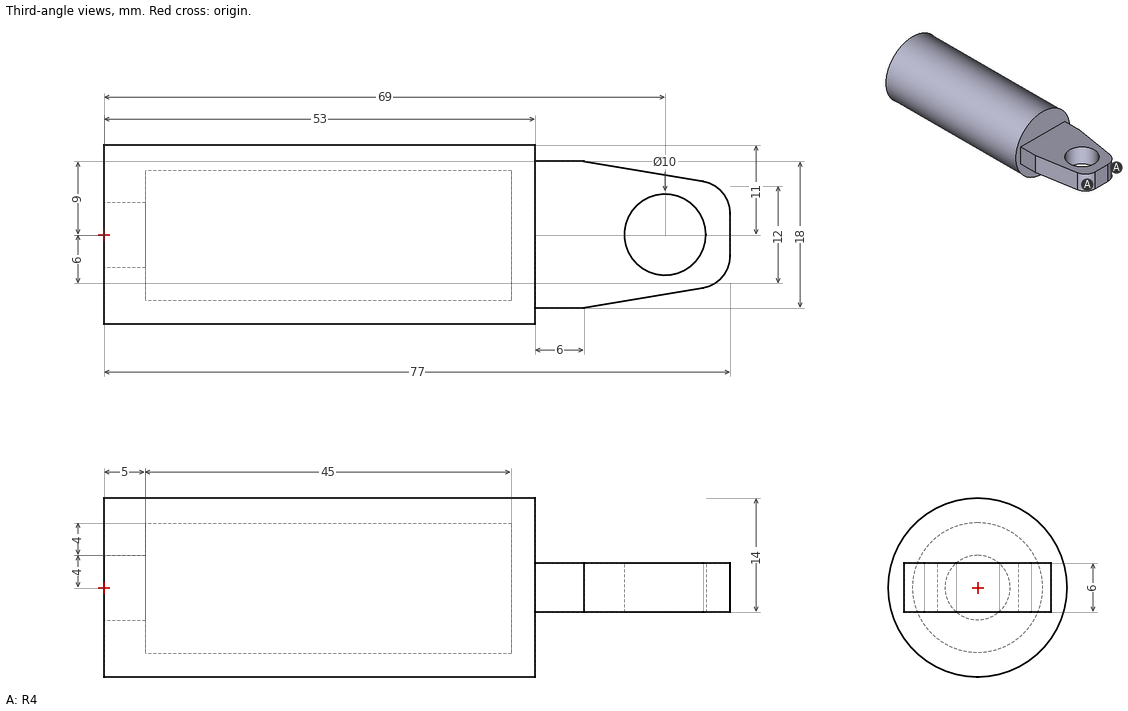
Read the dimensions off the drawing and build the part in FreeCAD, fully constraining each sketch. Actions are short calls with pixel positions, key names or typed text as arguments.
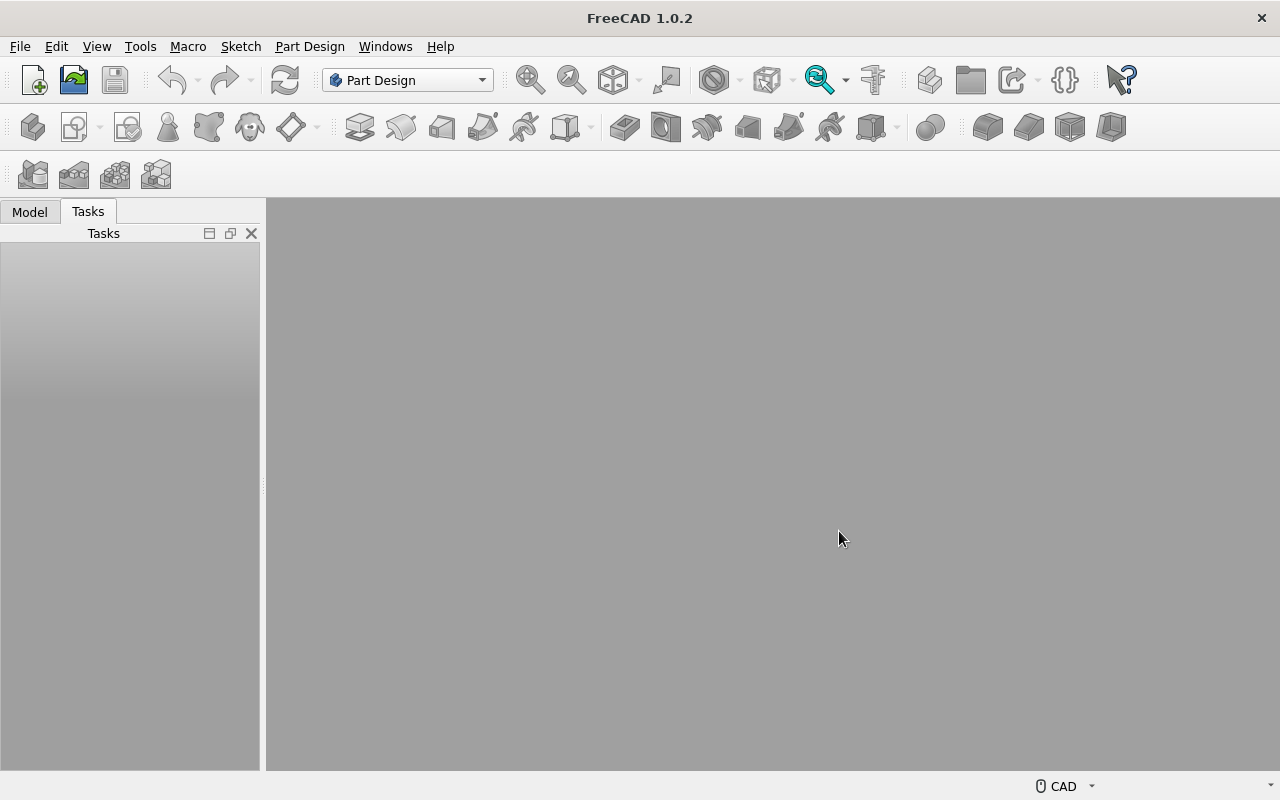
click(33, 80)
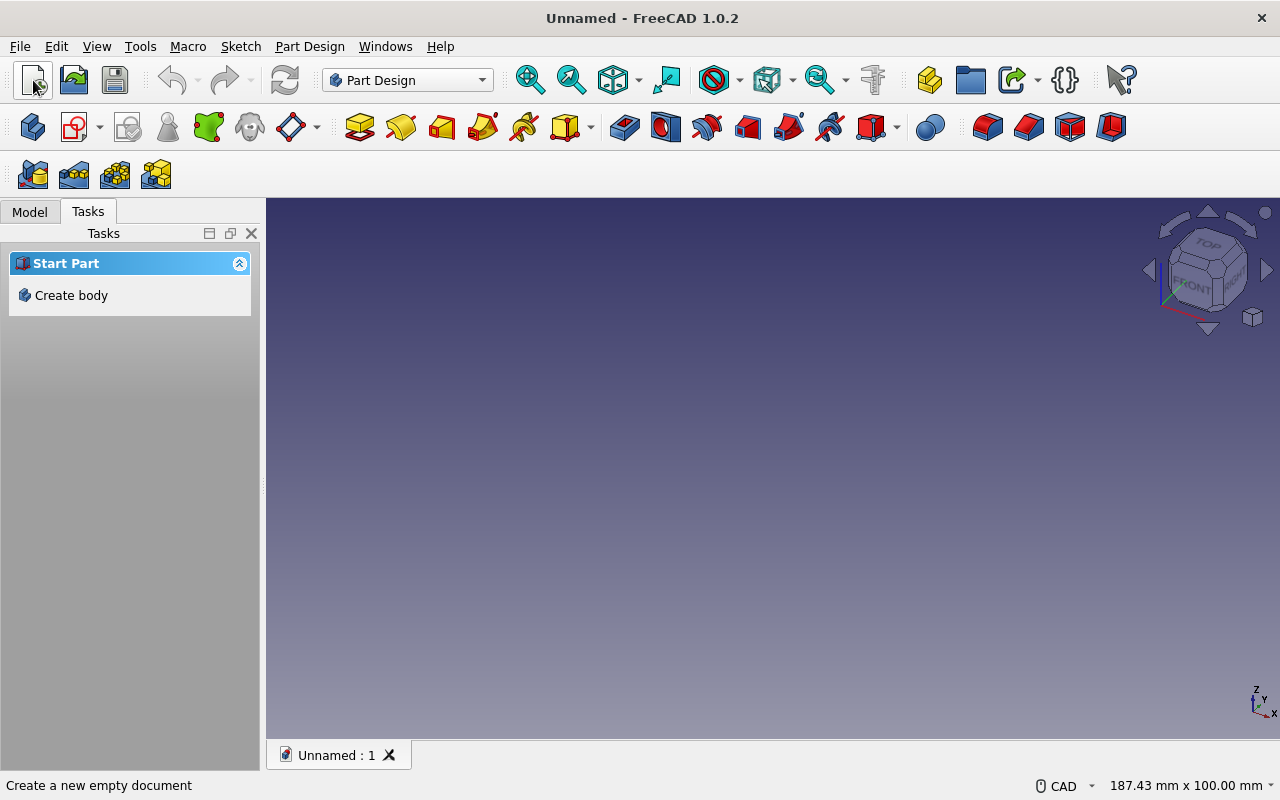
click(74, 128)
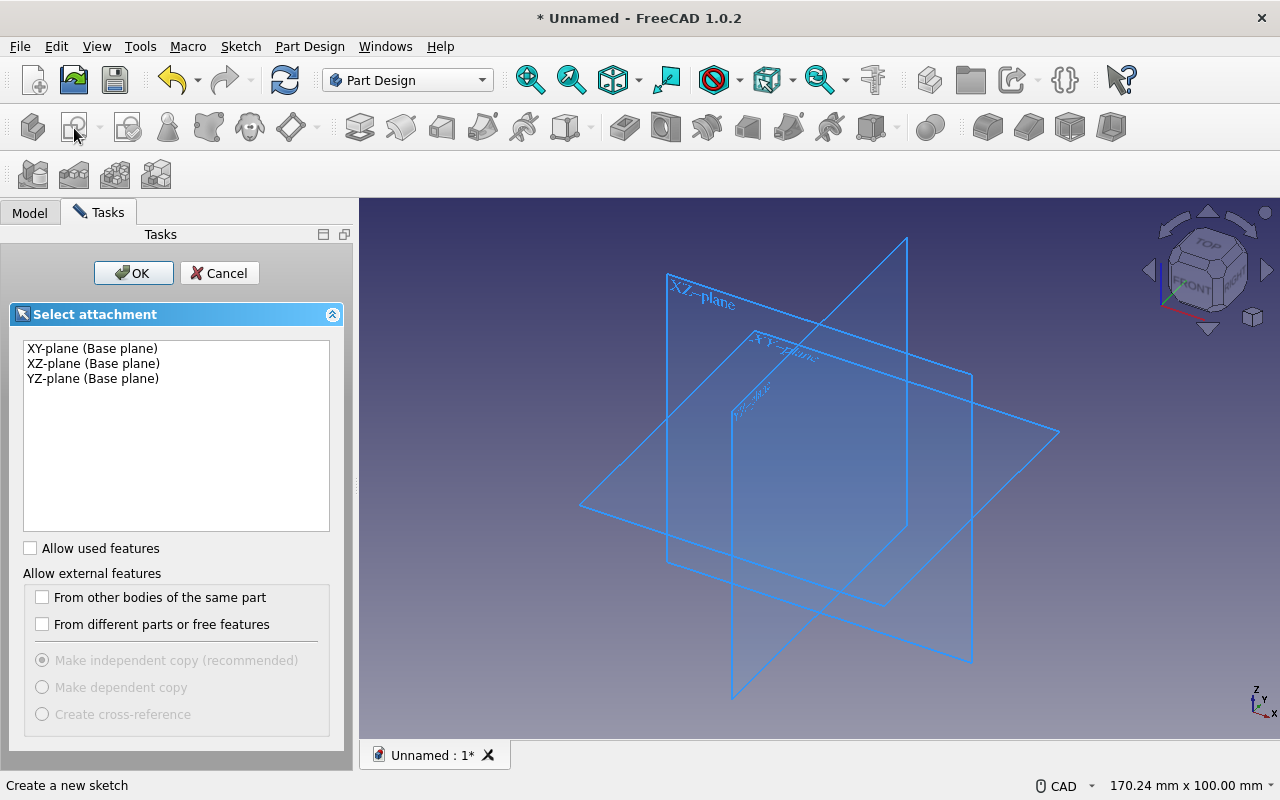
click(84, 348)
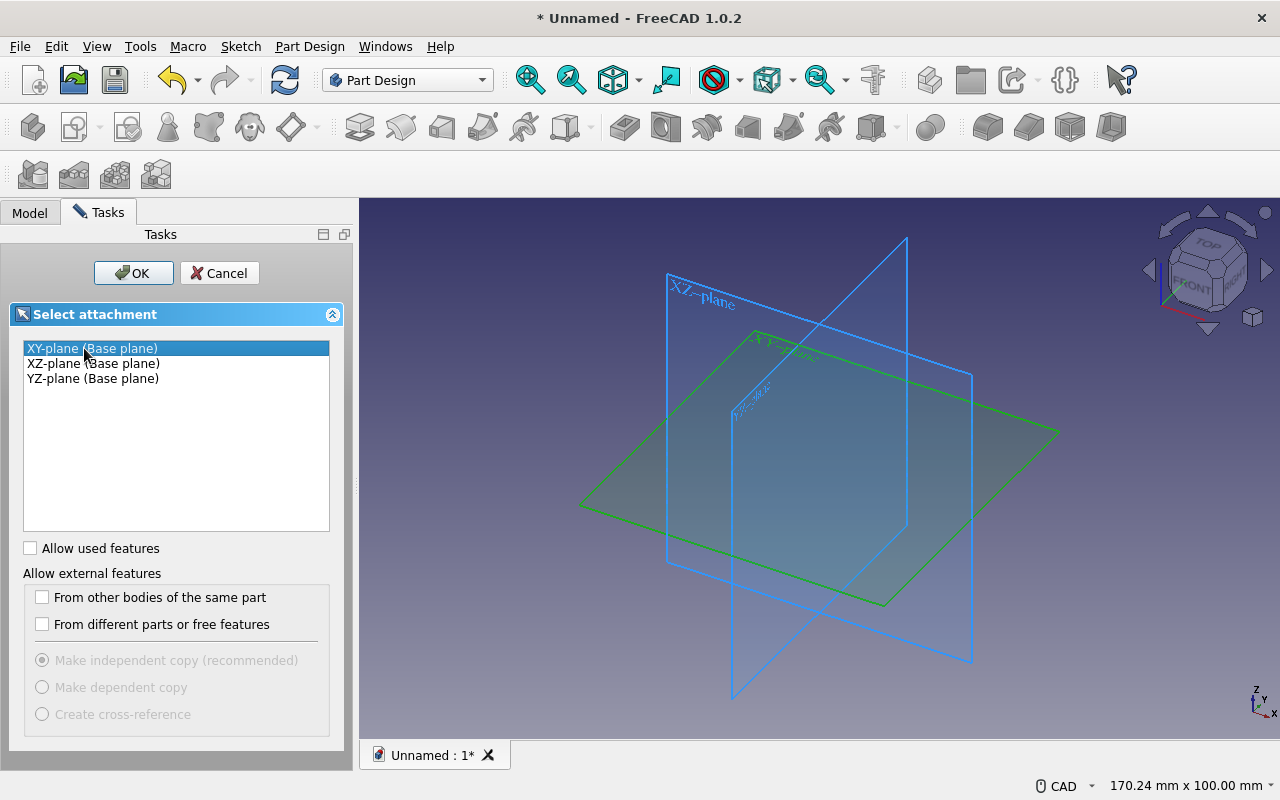
click(134, 273)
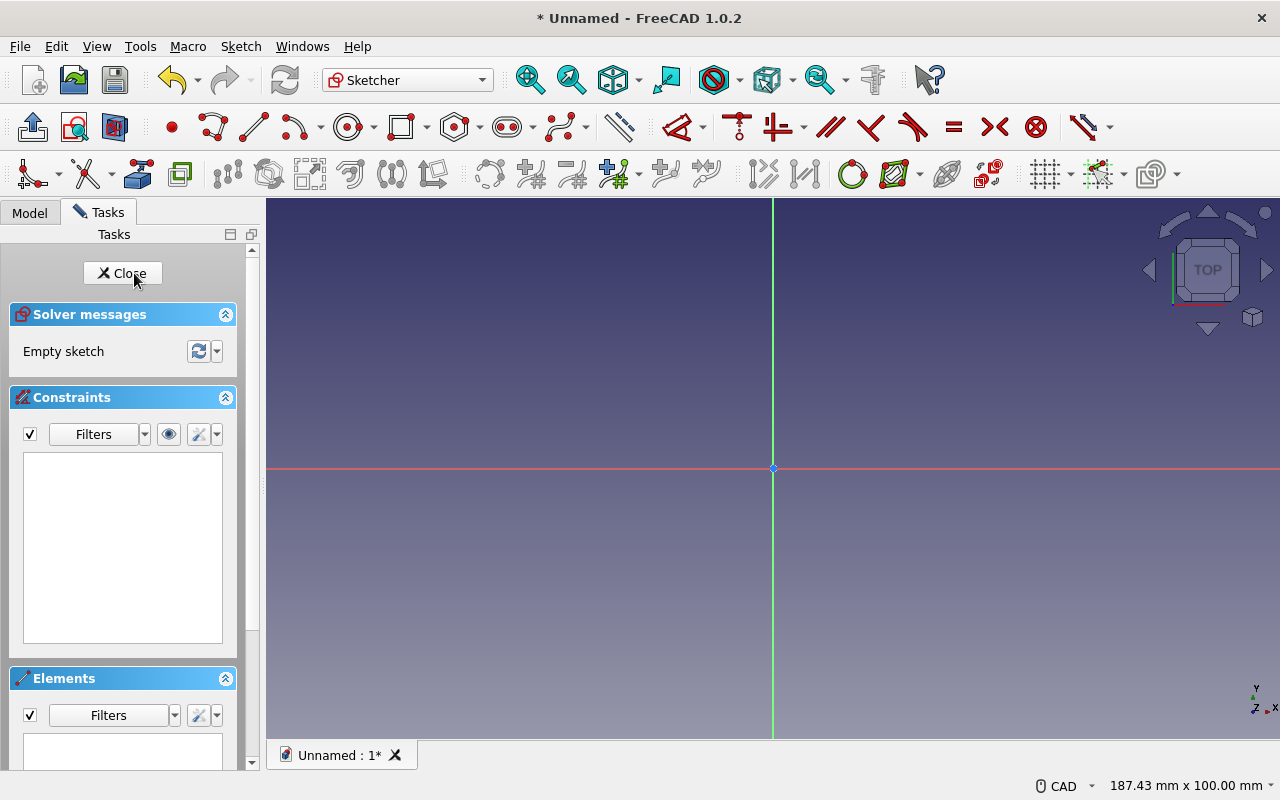
scroll(1089, 414, up, 4)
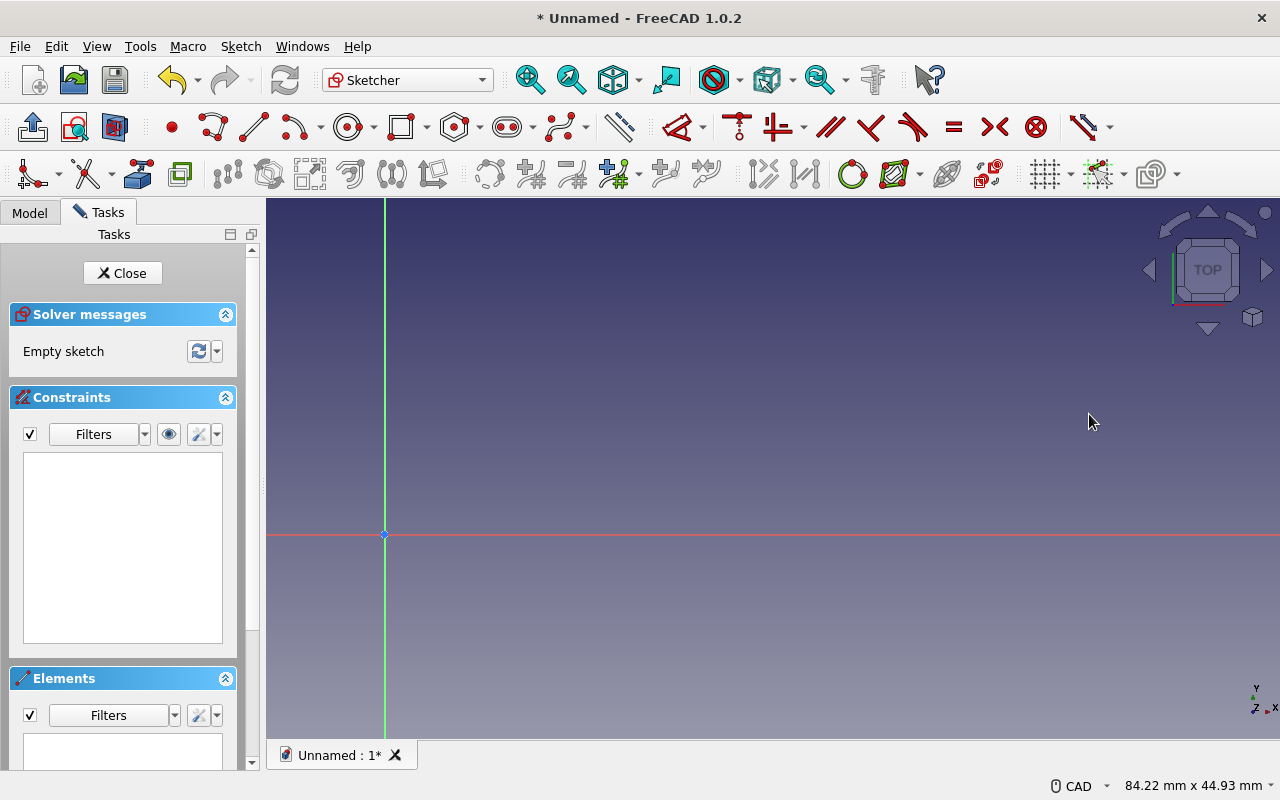
click(400, 128)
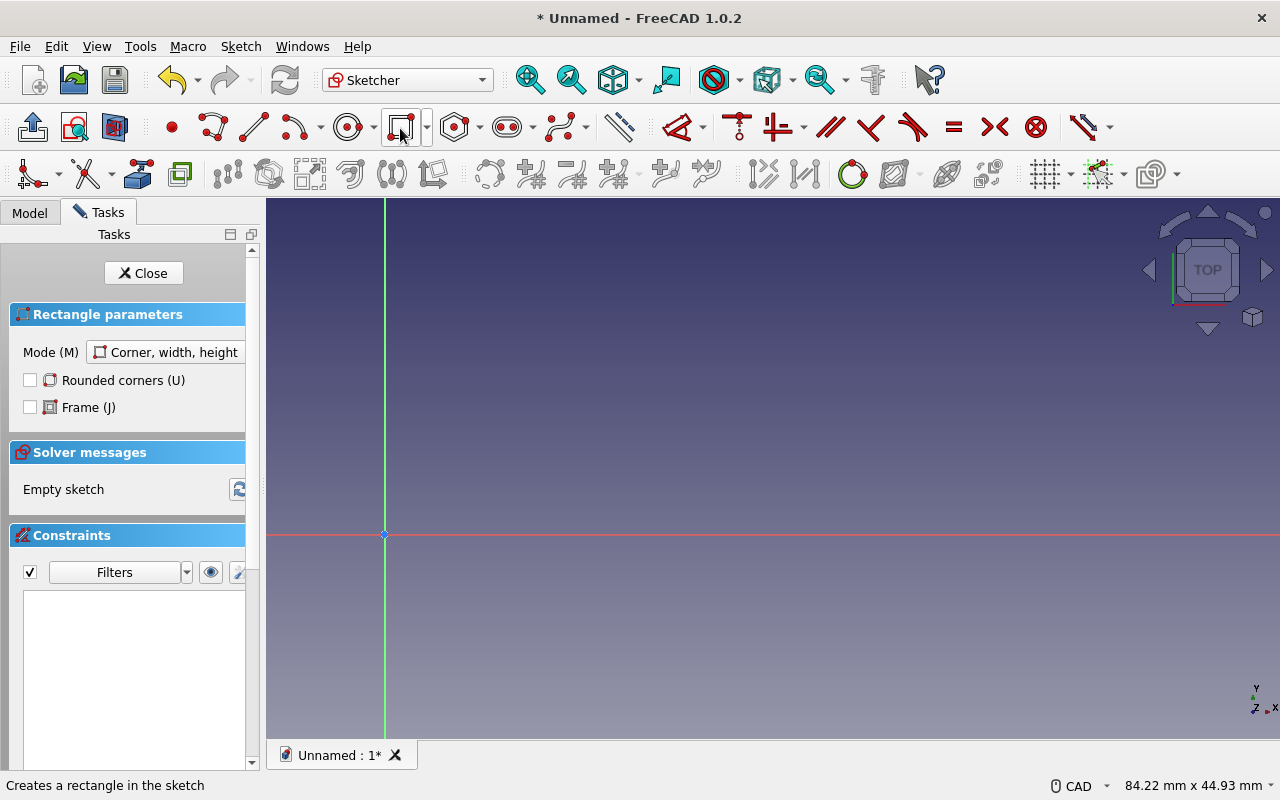
click(385, 535)
click(1023, 402)
key(Escape)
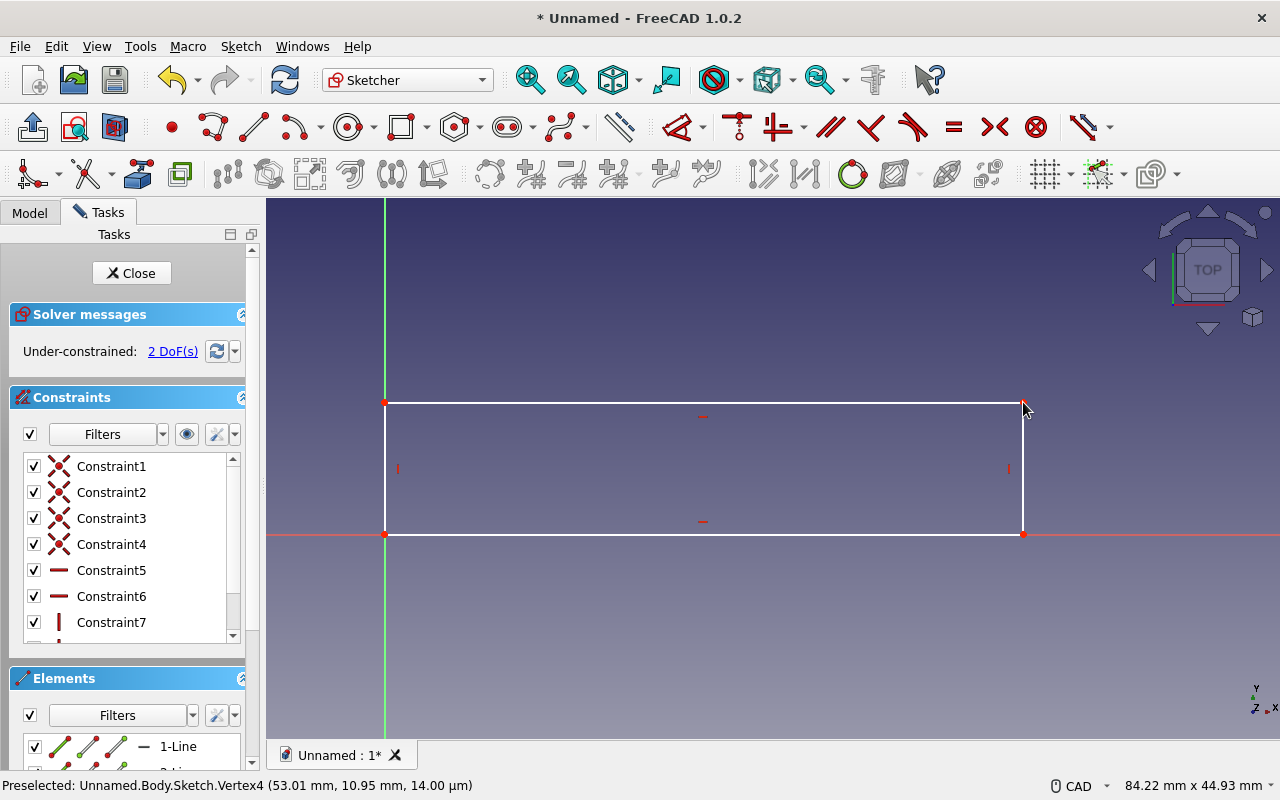
click(576, 535)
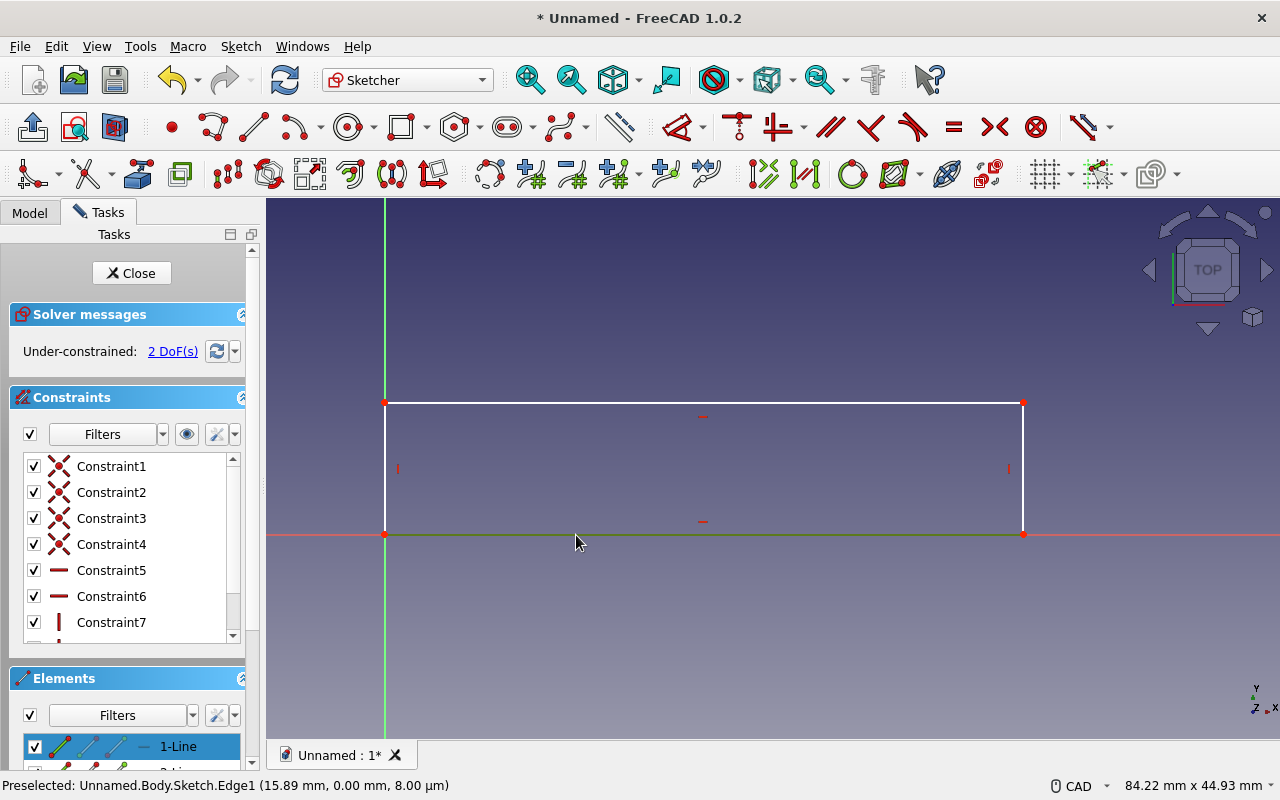
key(l)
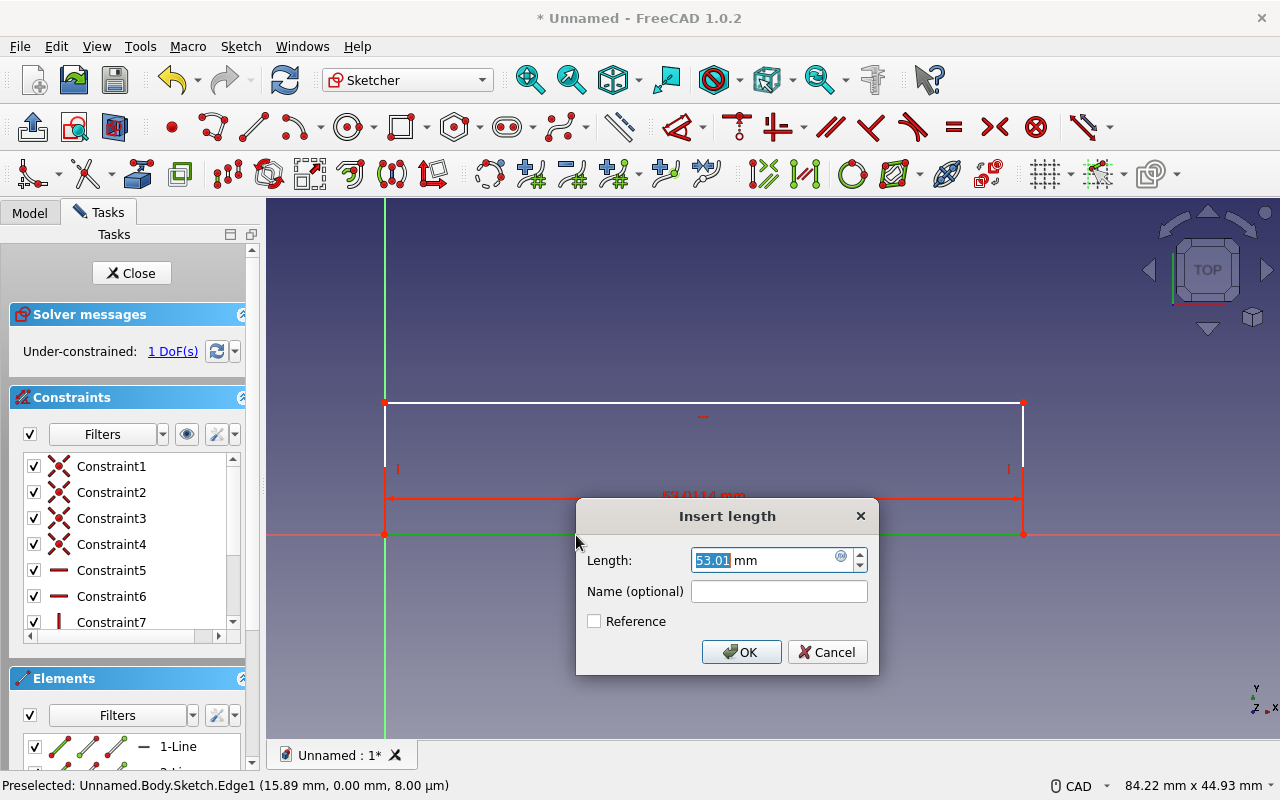
text(53)
key(Return)